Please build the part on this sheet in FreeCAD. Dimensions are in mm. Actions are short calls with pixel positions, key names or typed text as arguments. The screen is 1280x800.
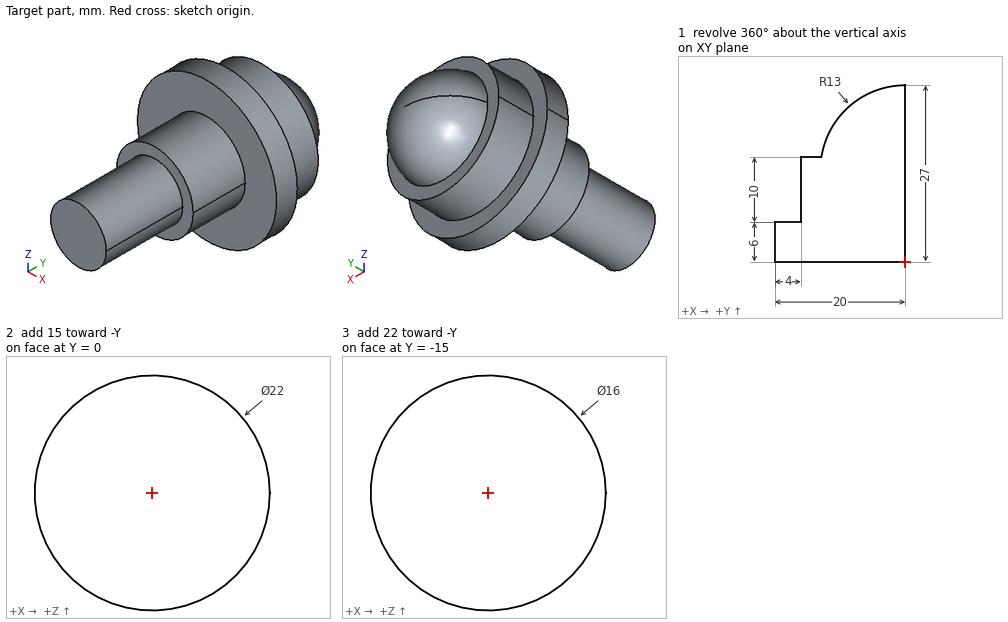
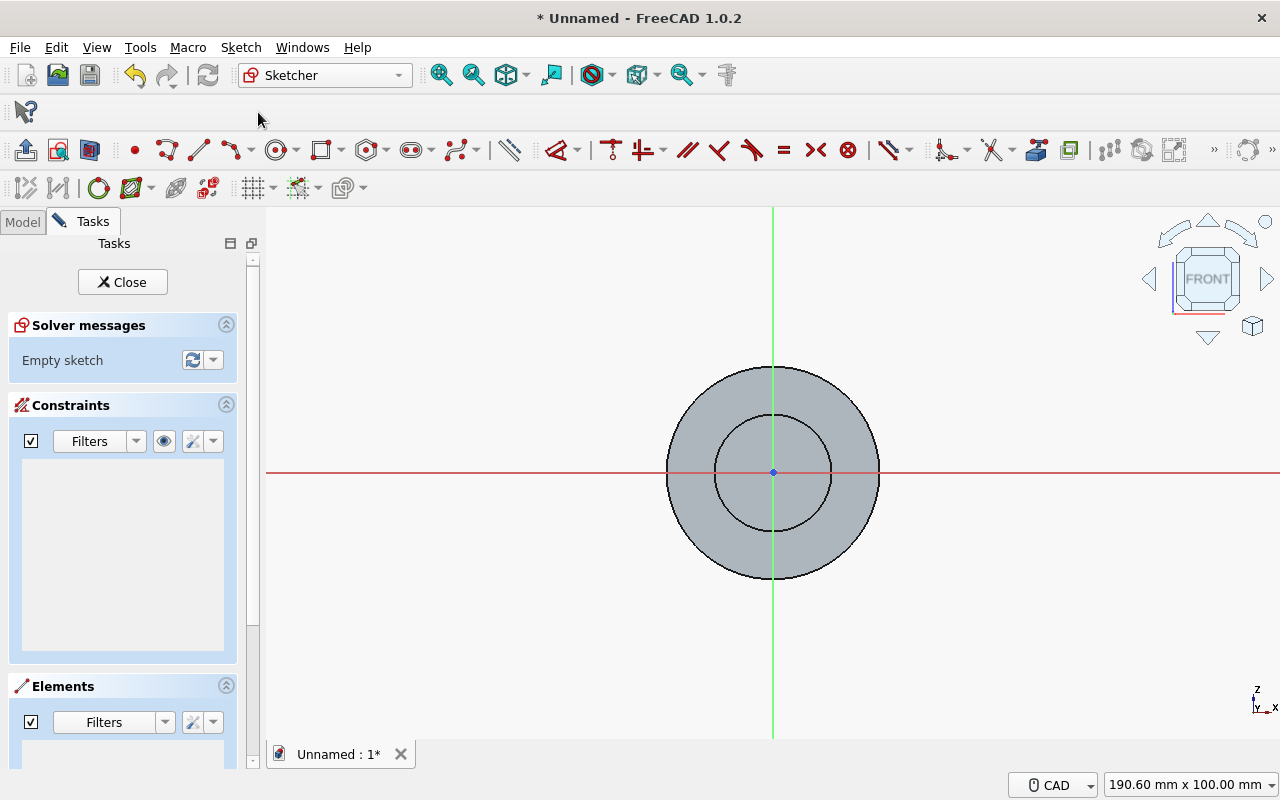
scroll(795, 473, up, 7)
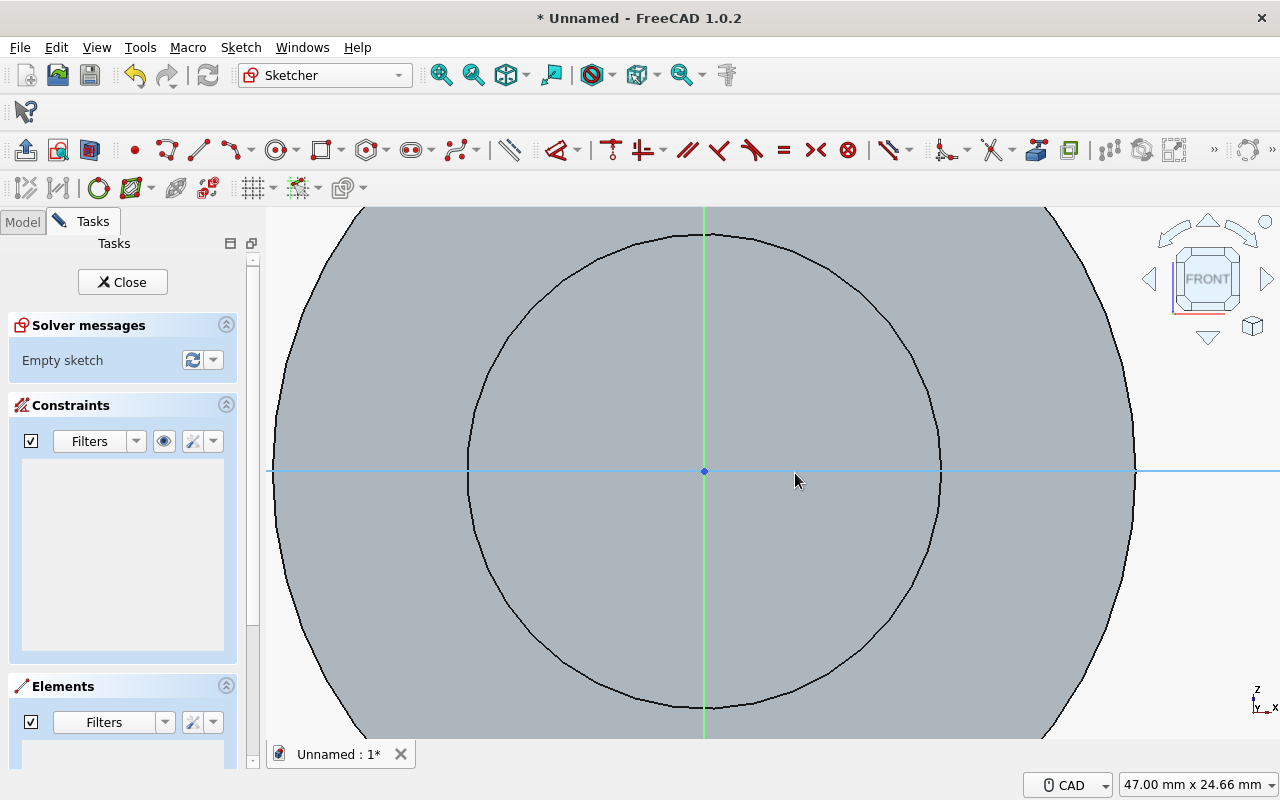
click(276, 150)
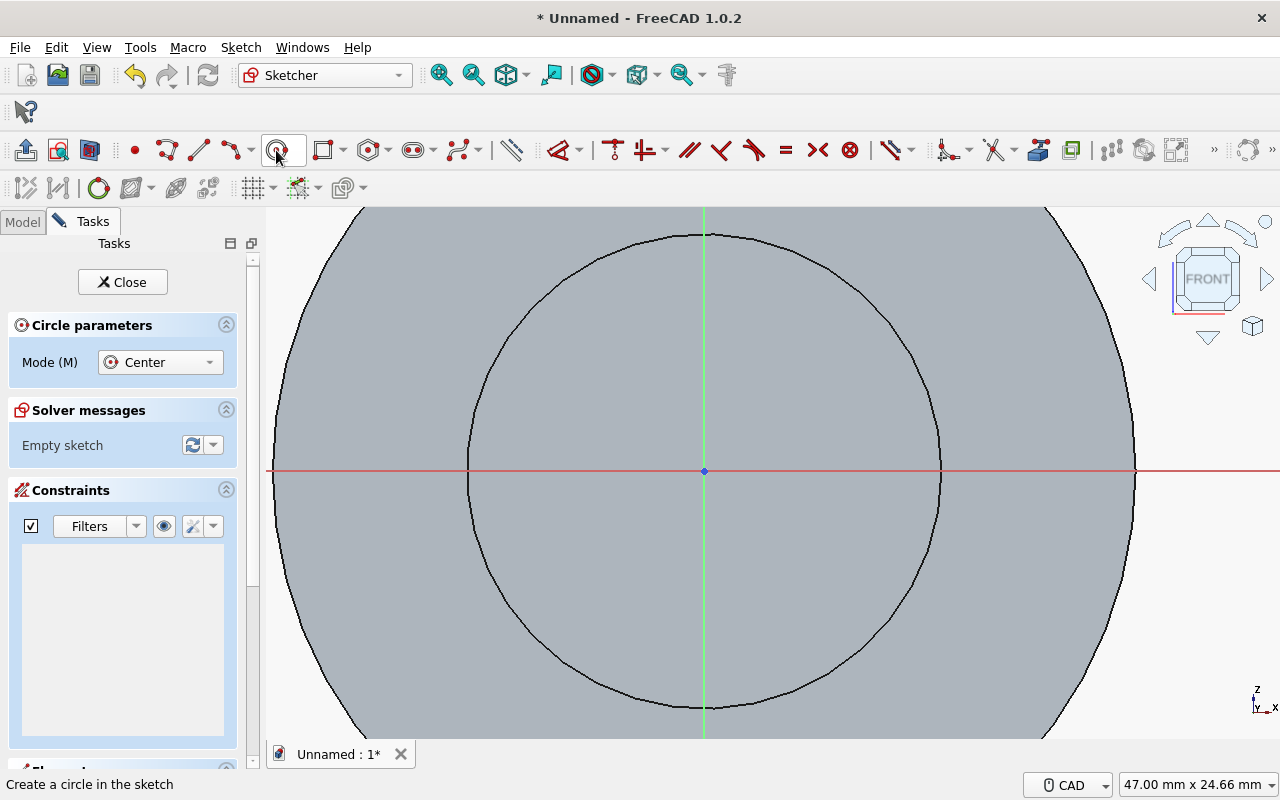
click(704, 471)
move(826, 349)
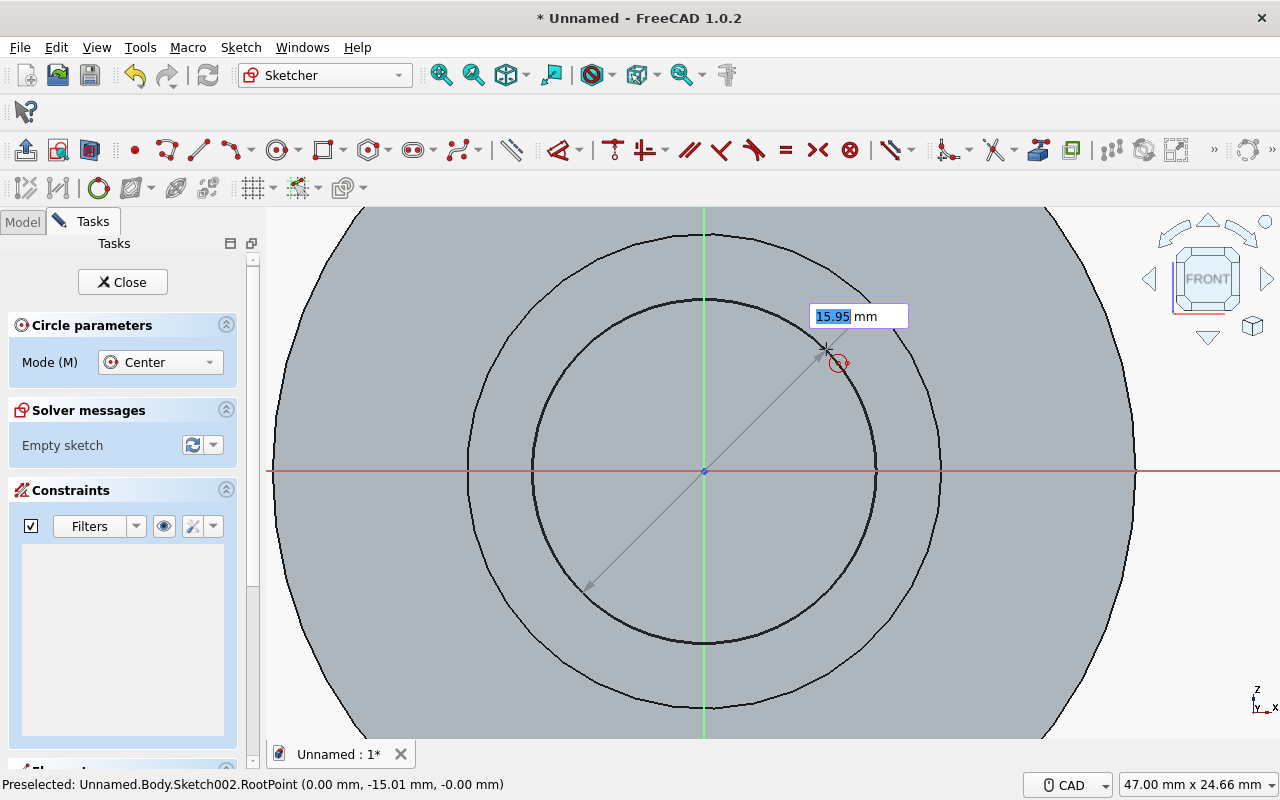
text(16)
key(Return)
key(Escape)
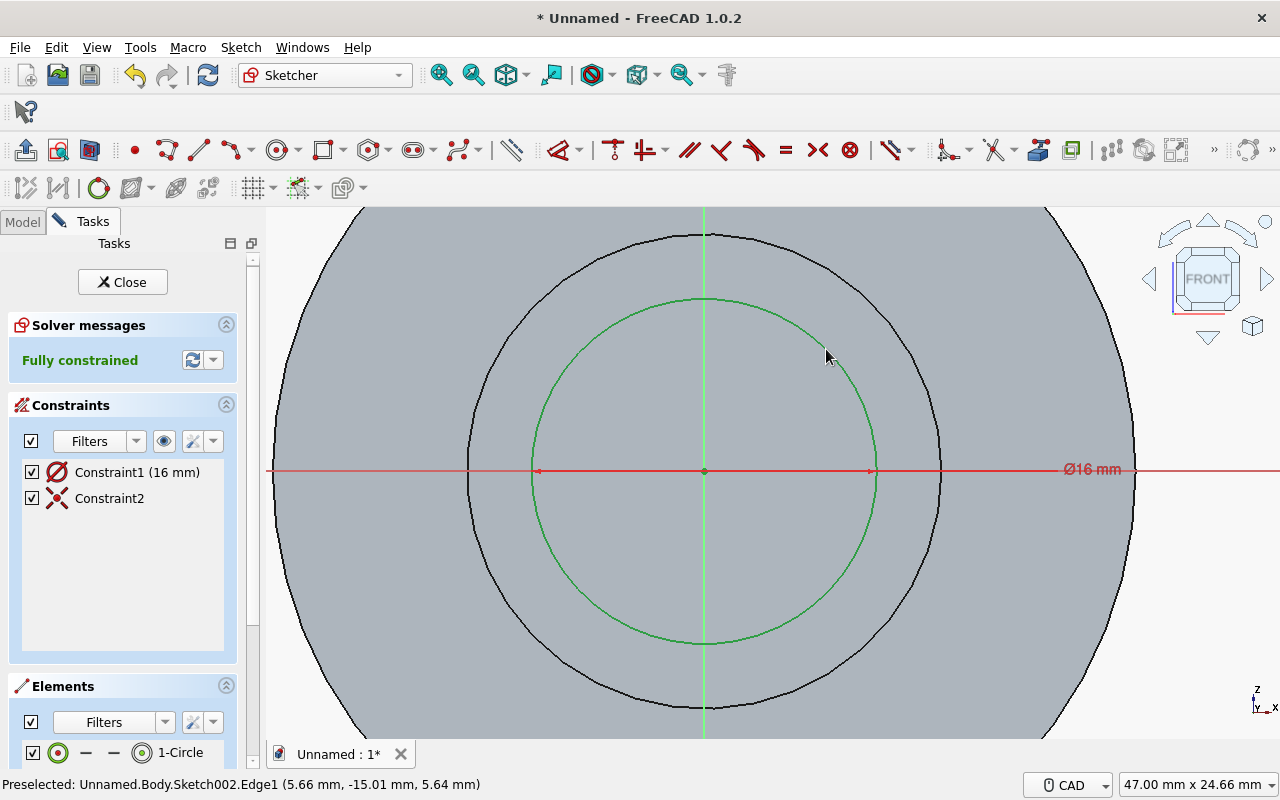
click(123, 282)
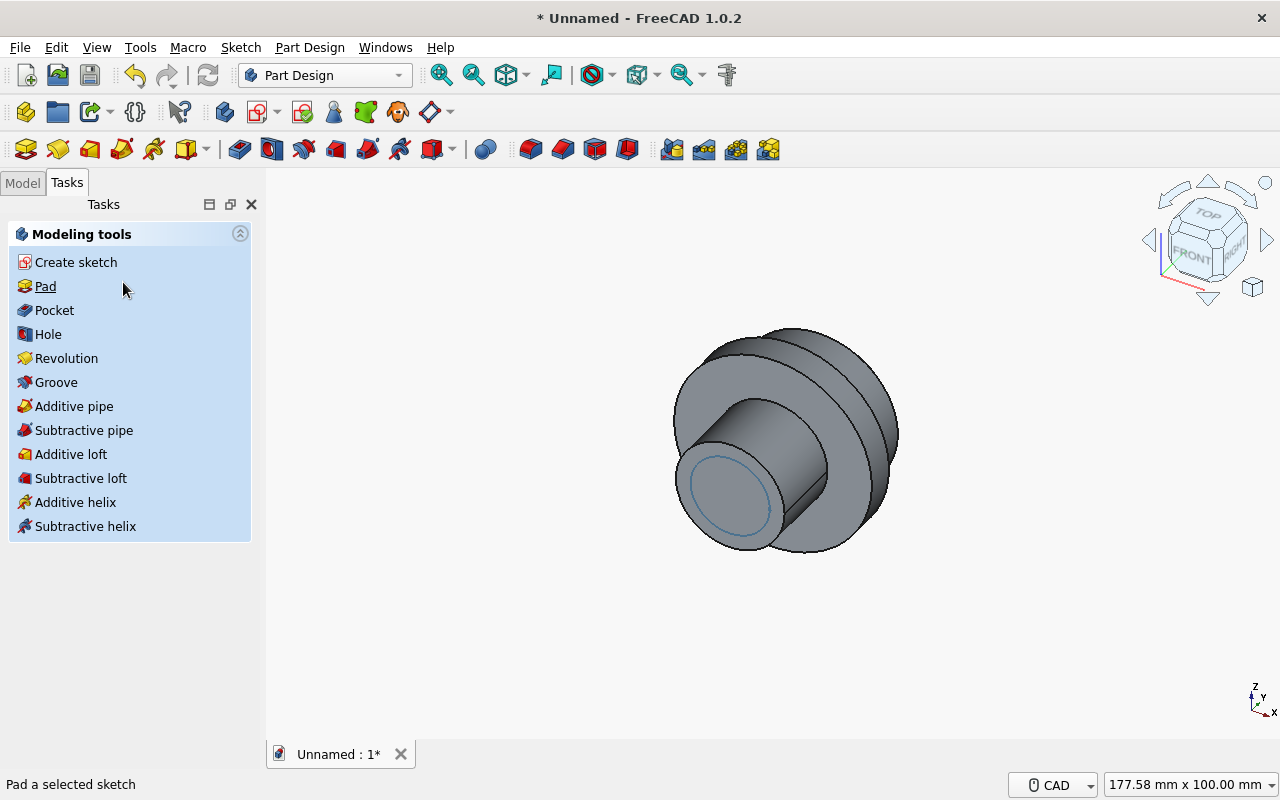
click(26, 150)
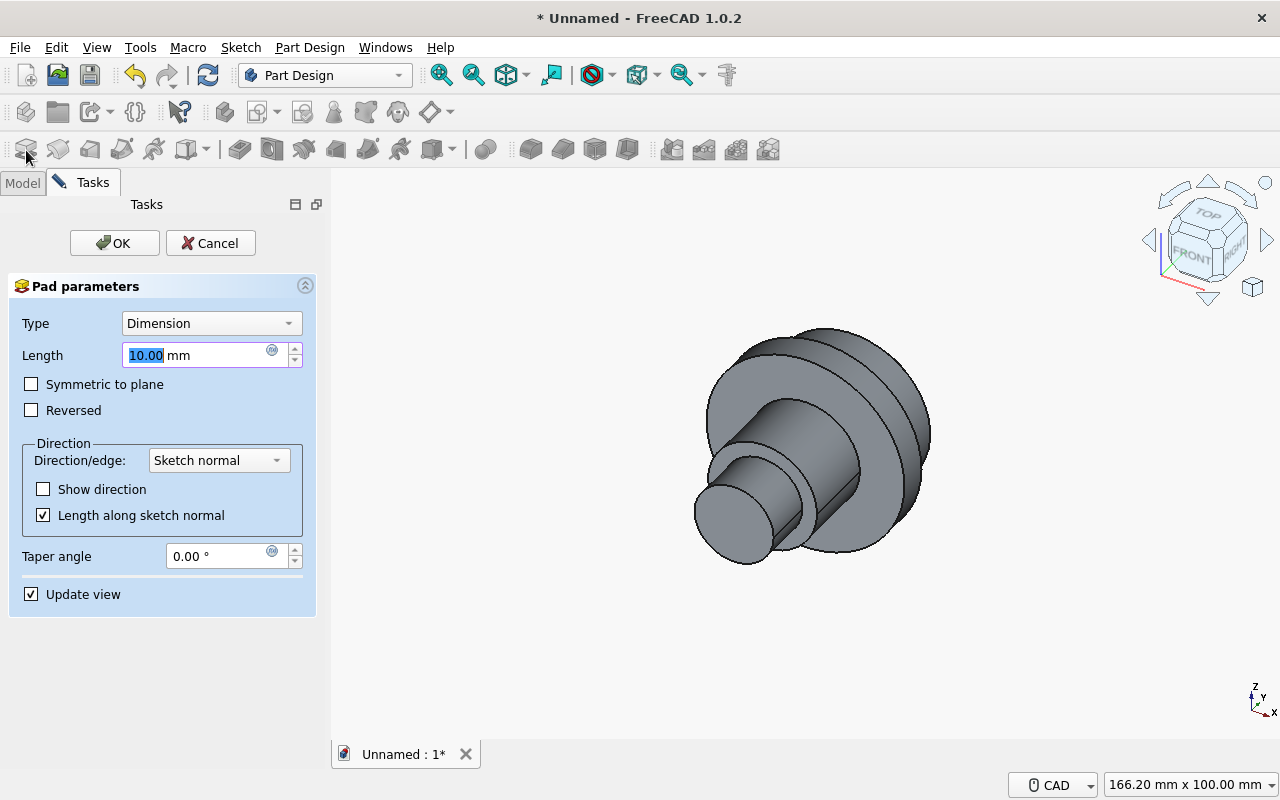
text(22)
key(Tab)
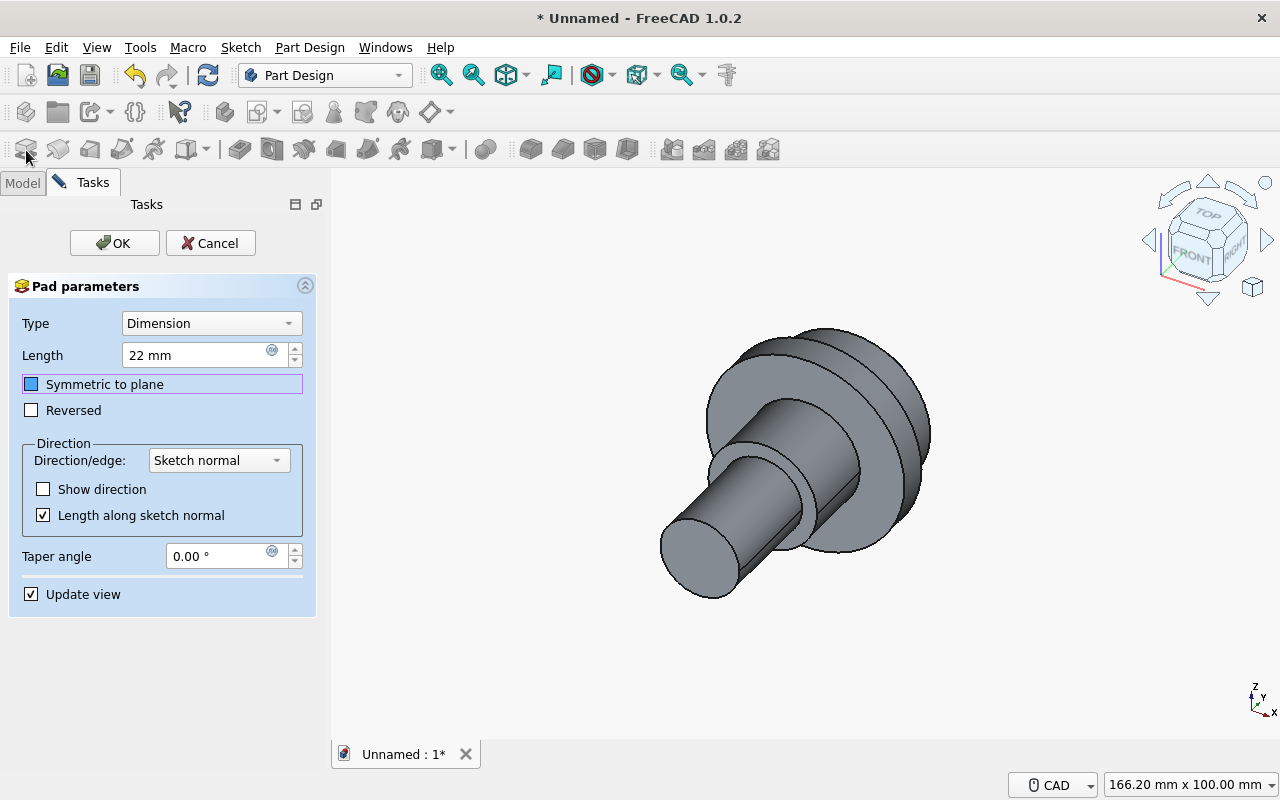
click(115, 243)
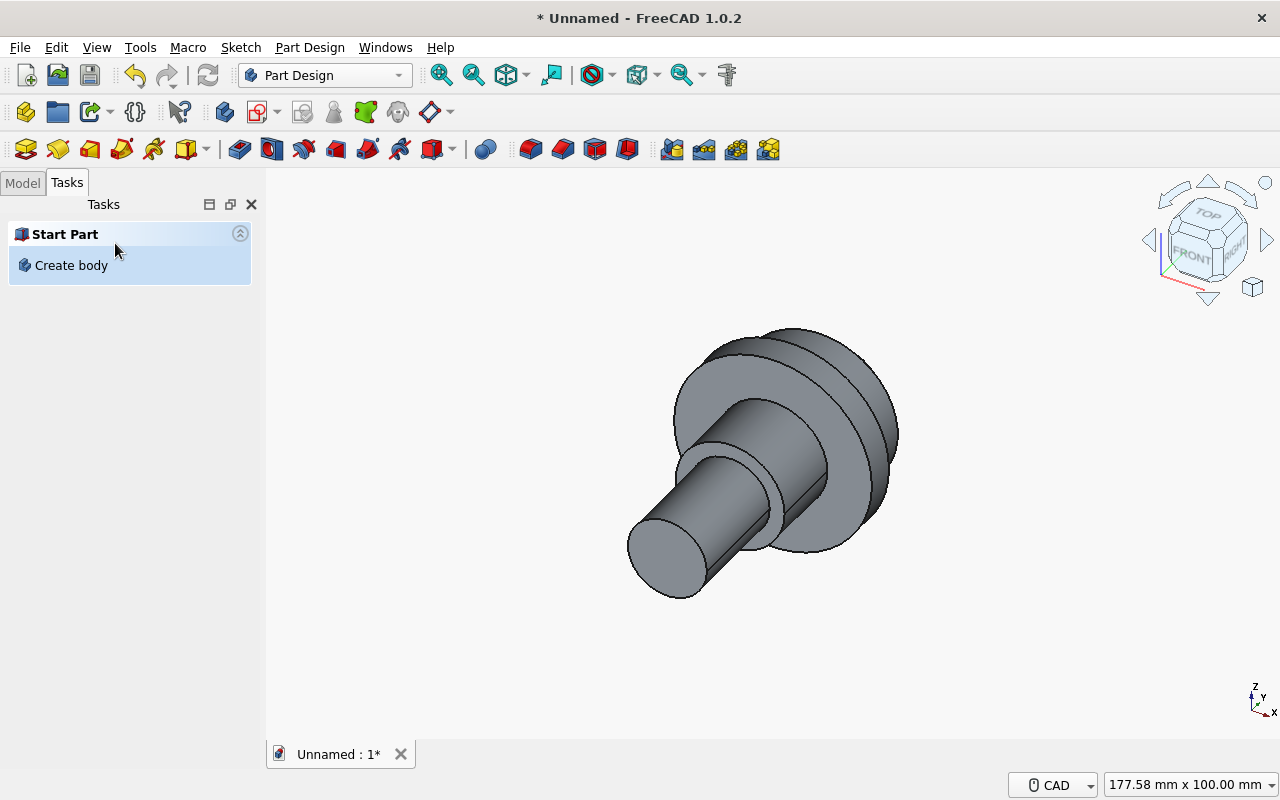
key(0)